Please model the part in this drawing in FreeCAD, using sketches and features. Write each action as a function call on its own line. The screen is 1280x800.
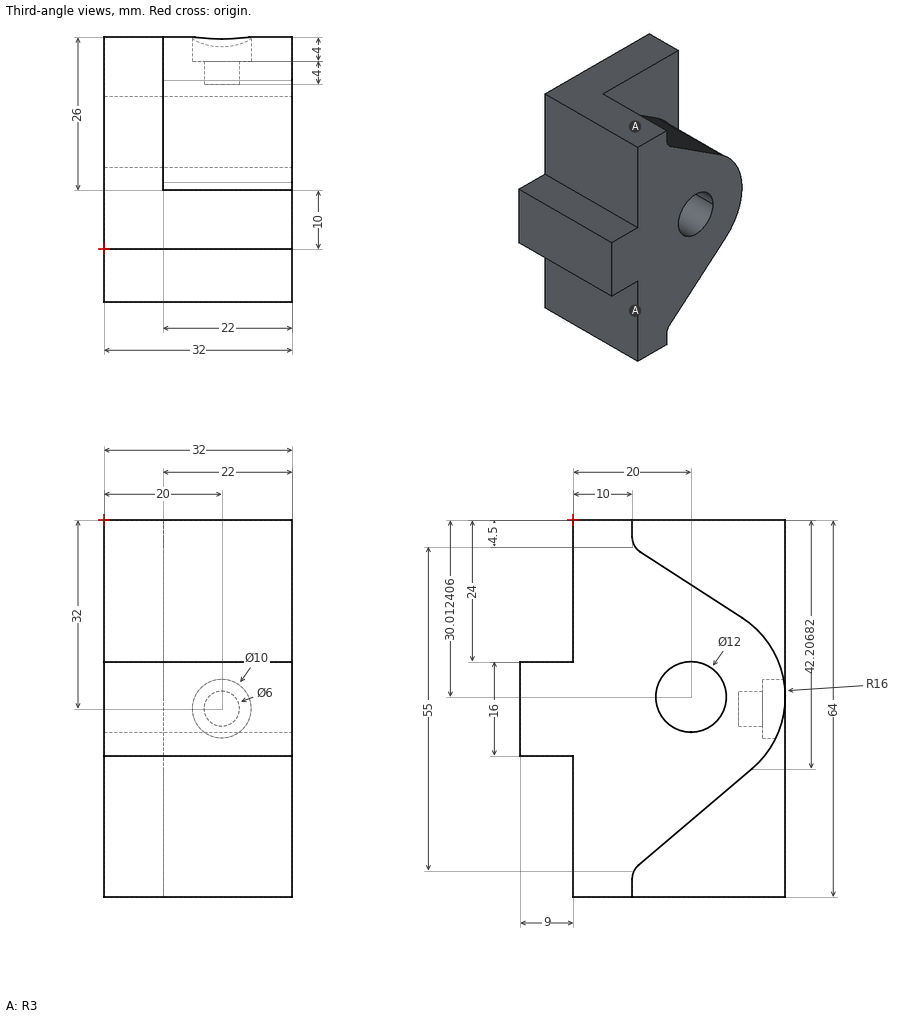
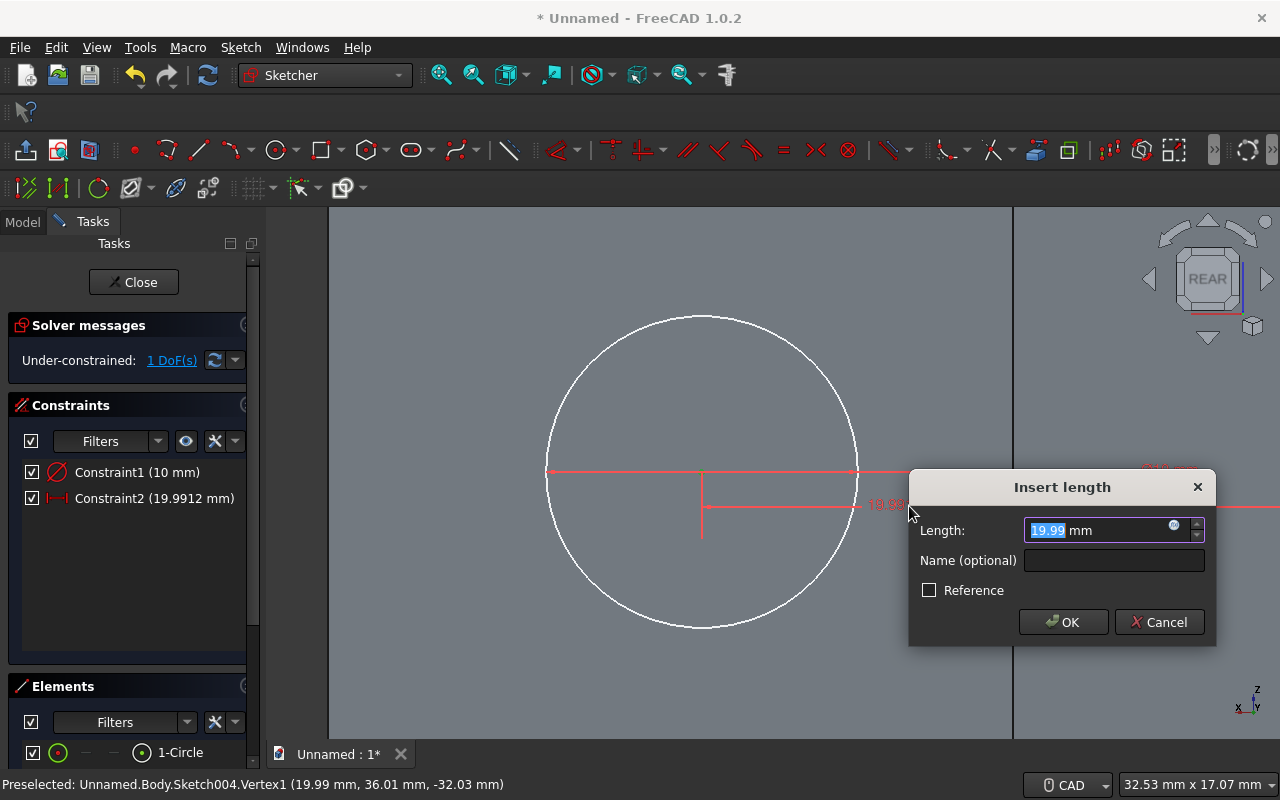
text(20)
key(Return)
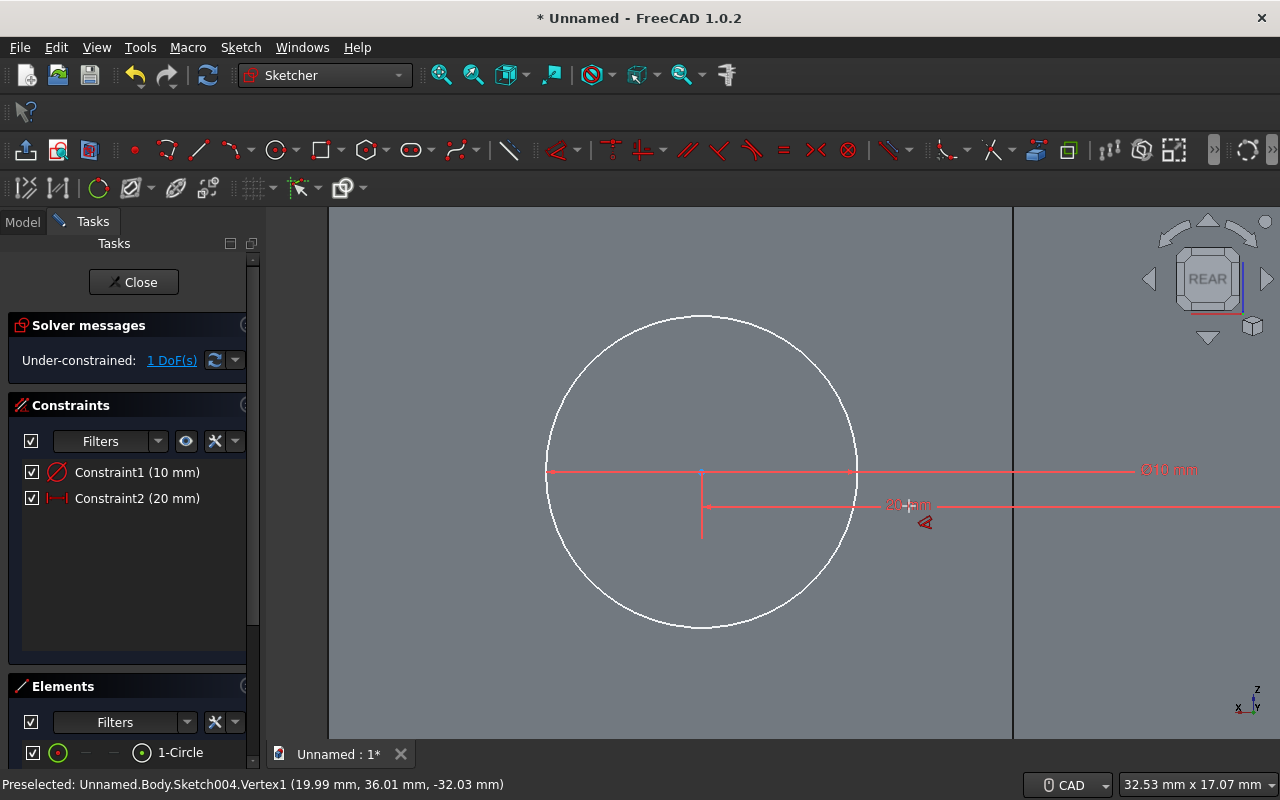
click(702, 472)
click(668, 354)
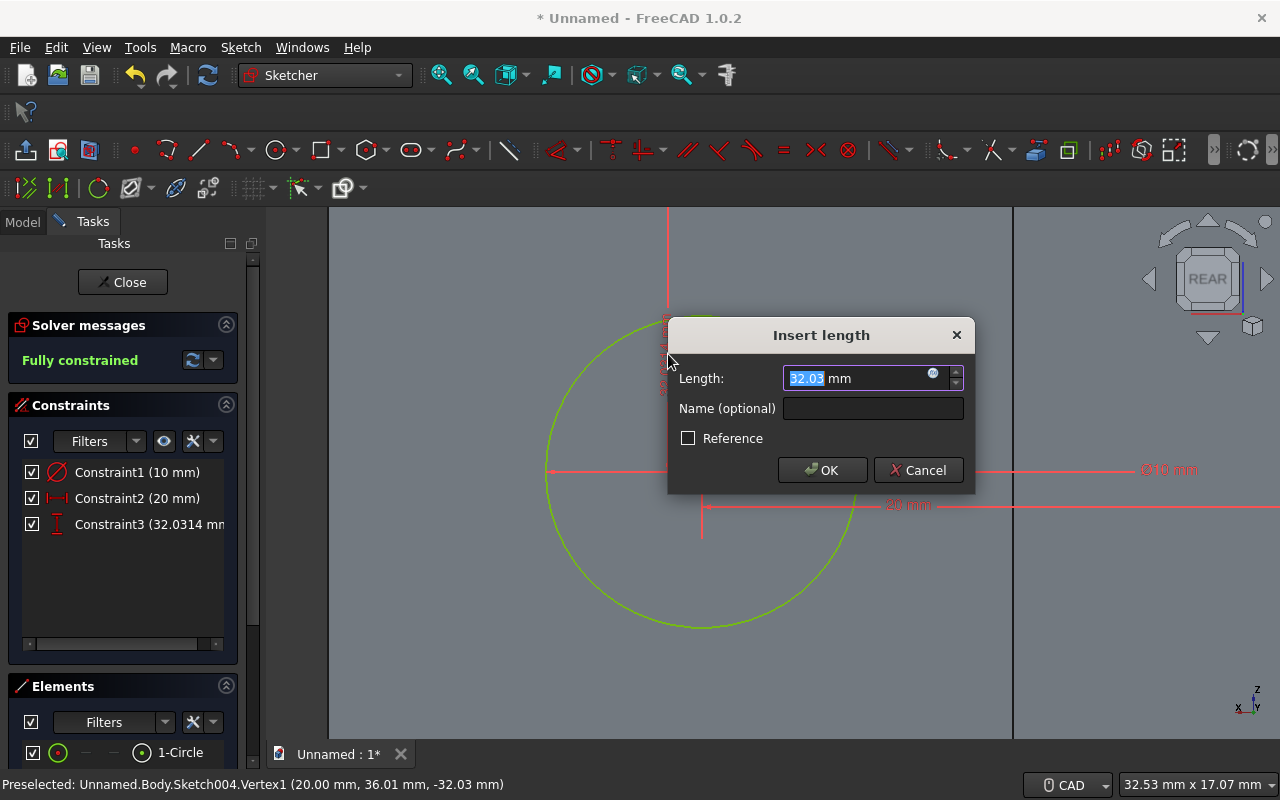
text(32)
key(Return)
key(Escape)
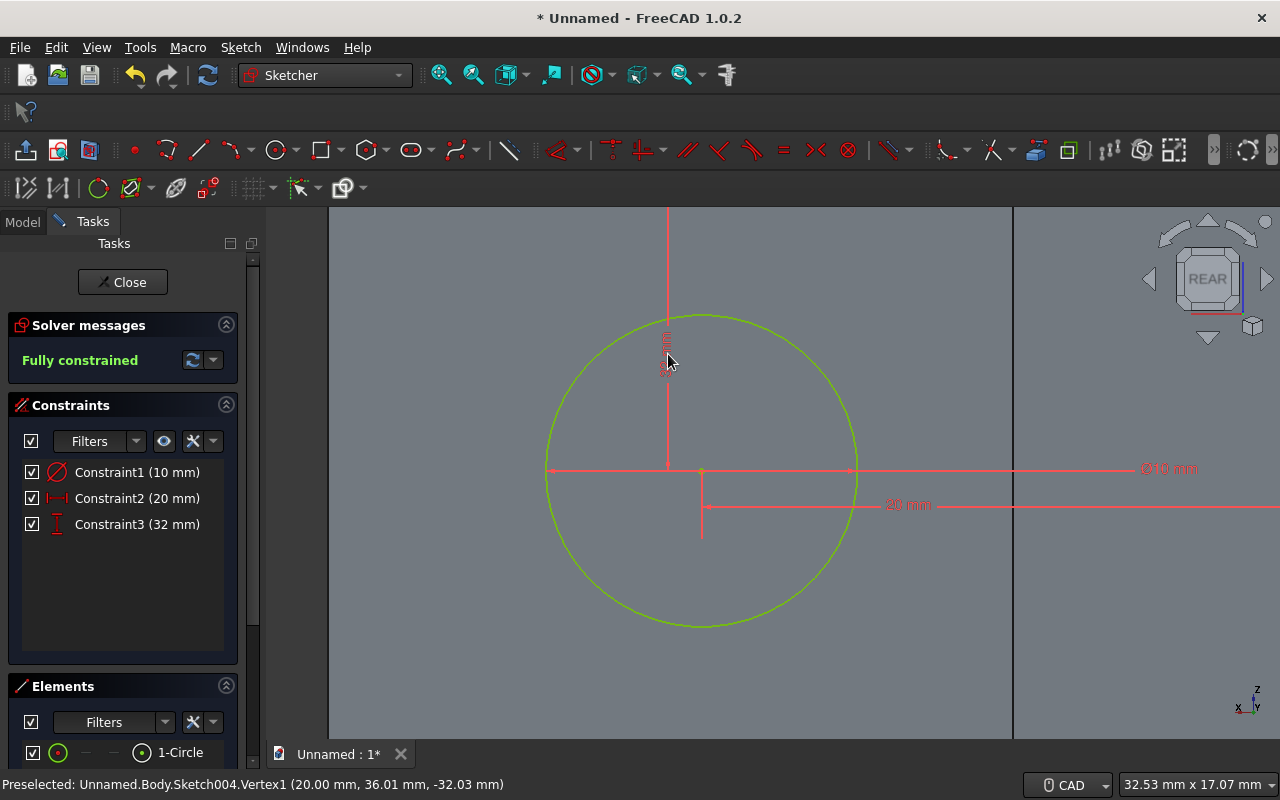
click(123, 282)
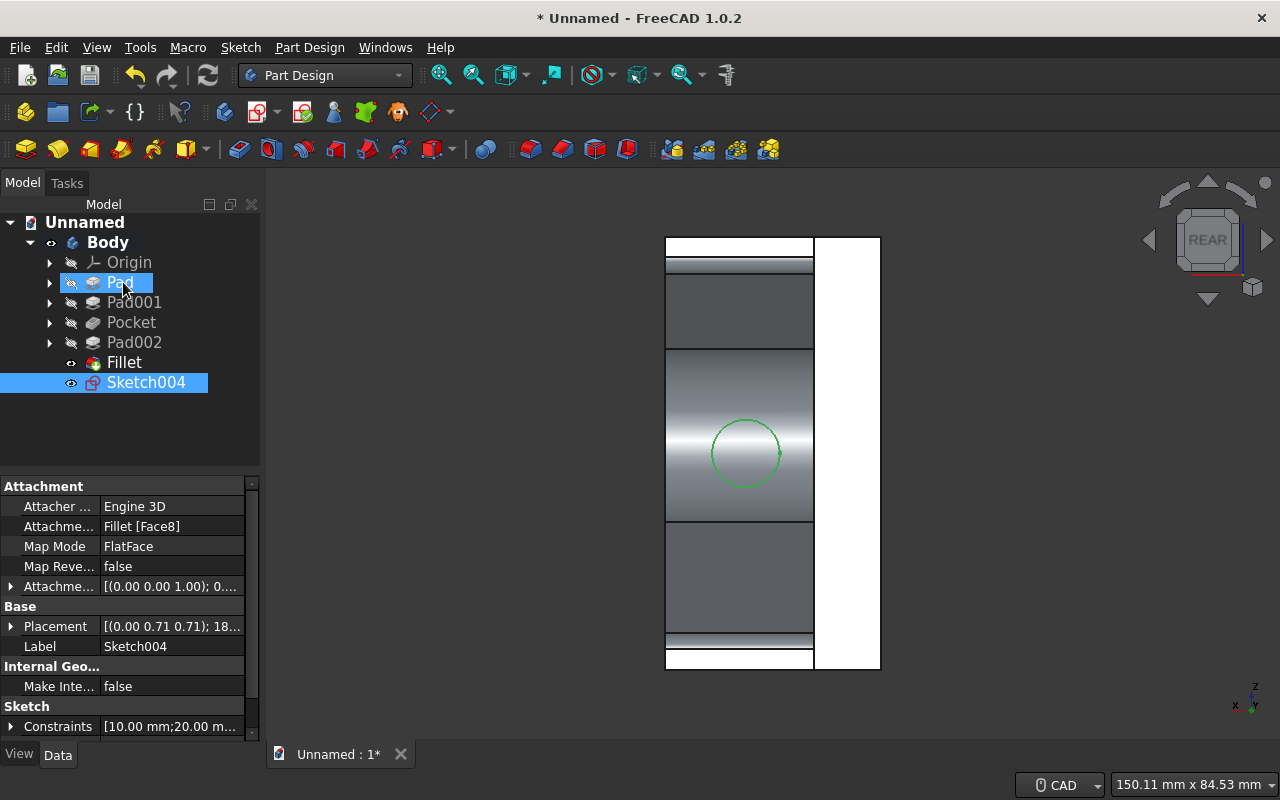
click(240, 150)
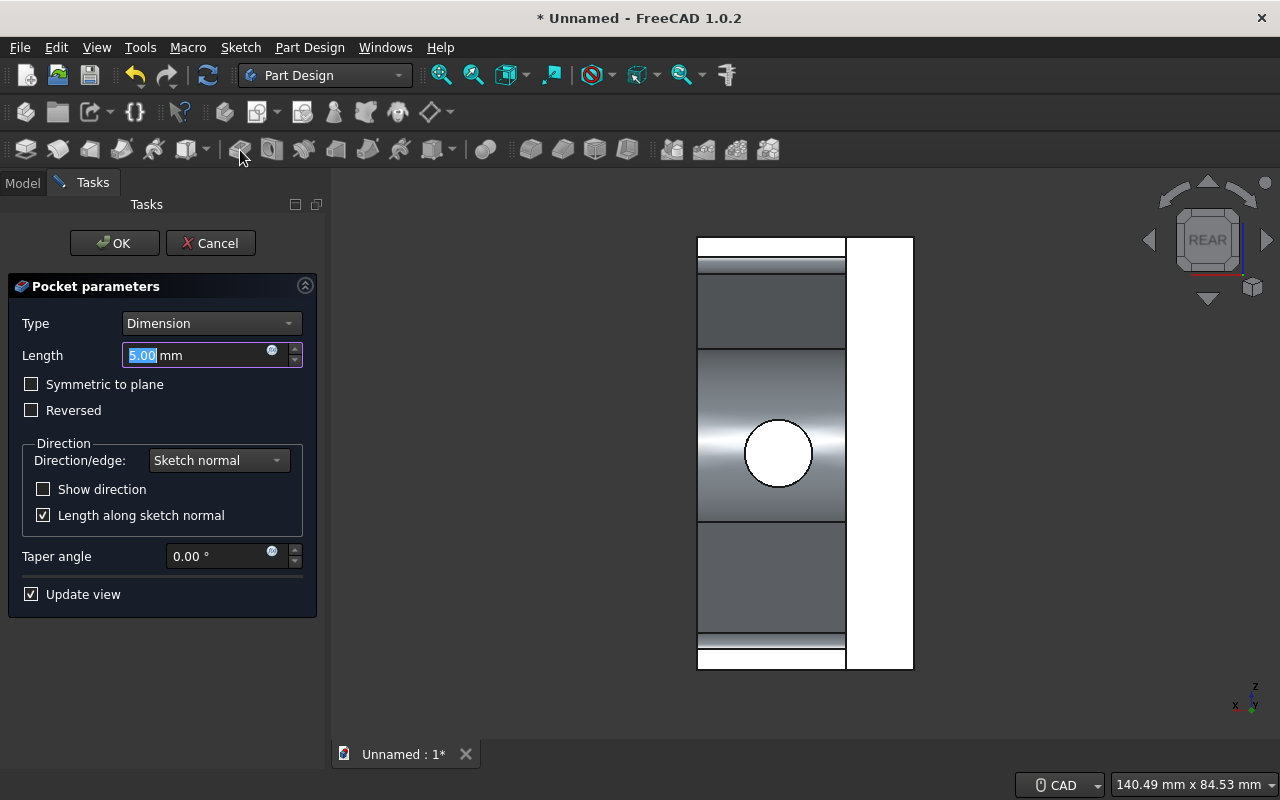
text(4)
key(Tab)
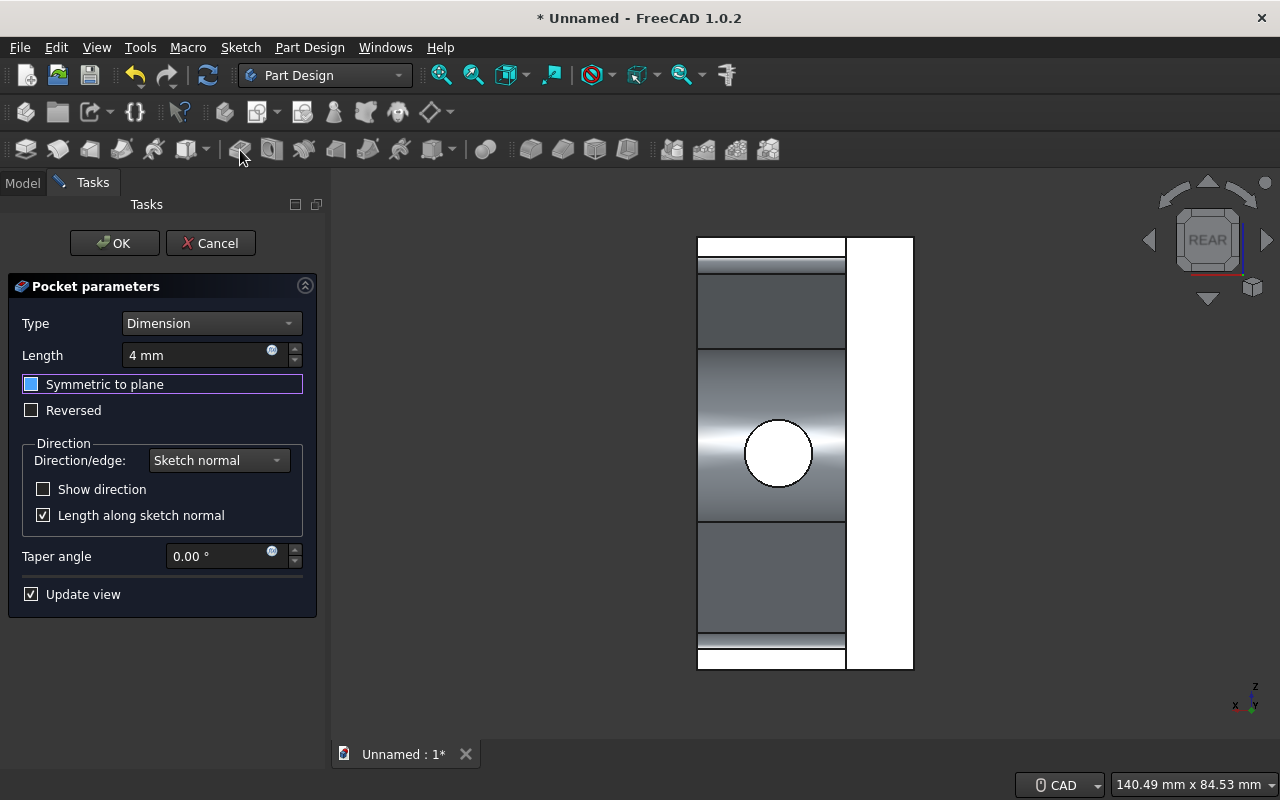
click(115, 243)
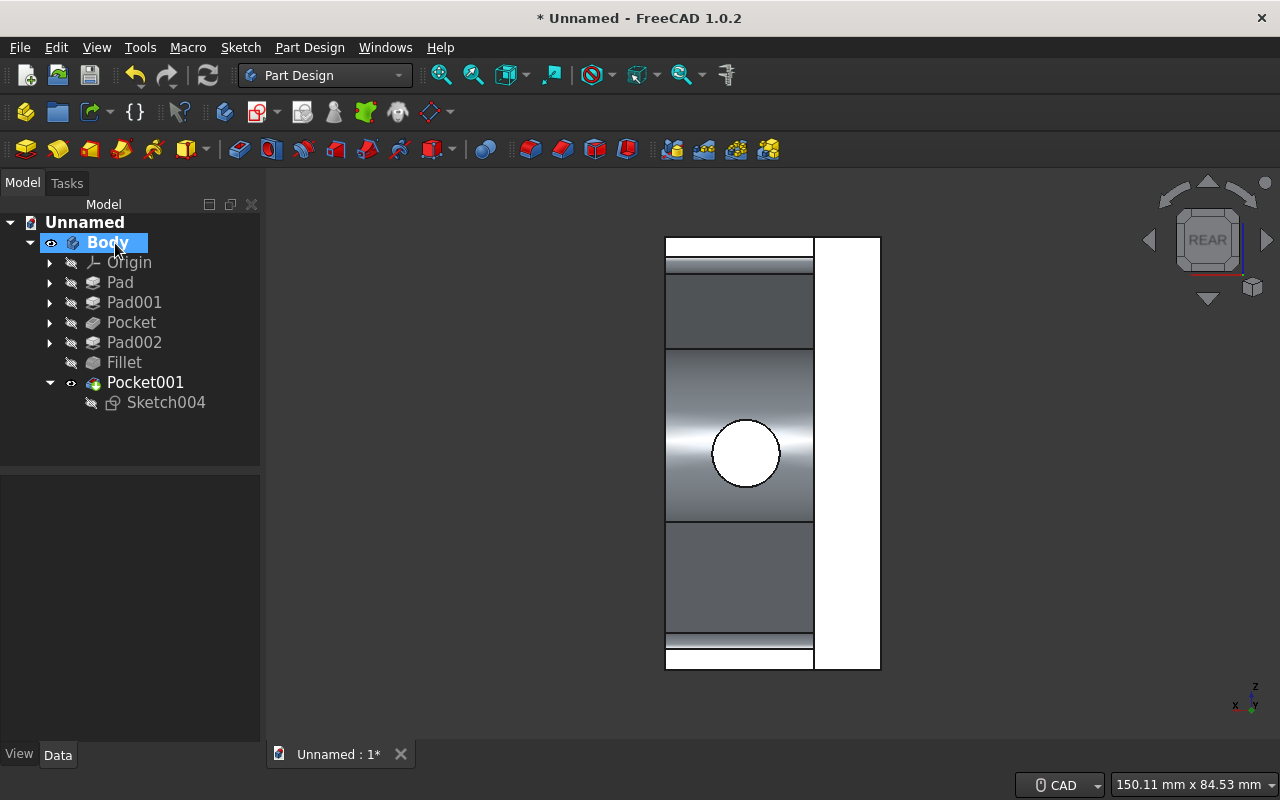
click(746, 453)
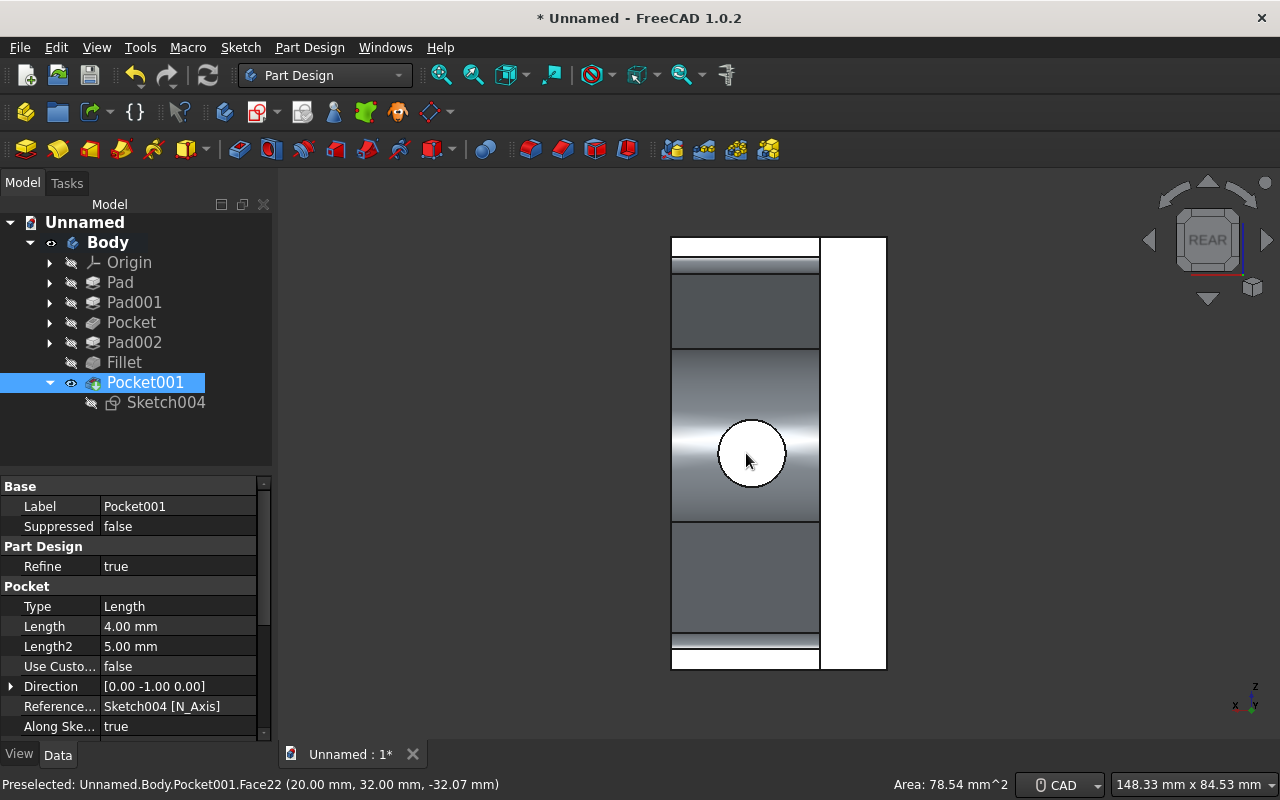
click(258, 112)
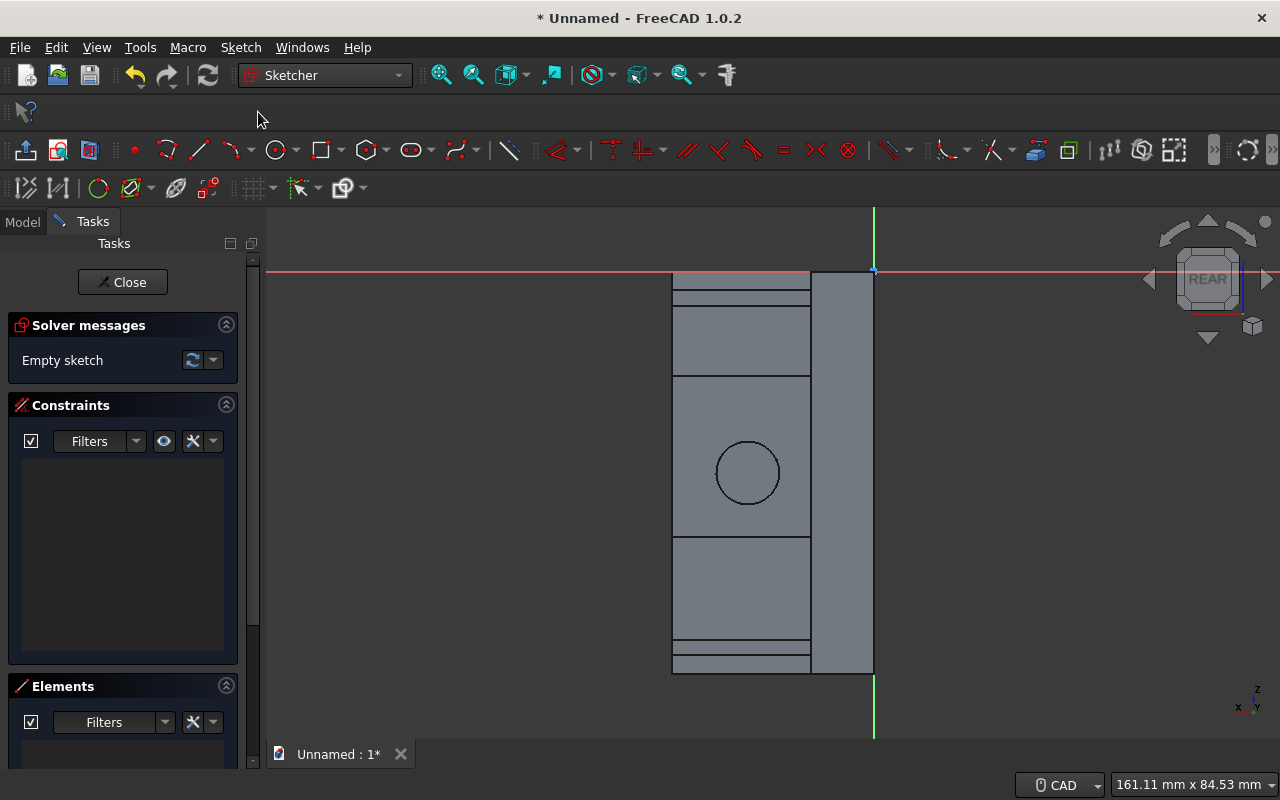
key(q)
key(s)